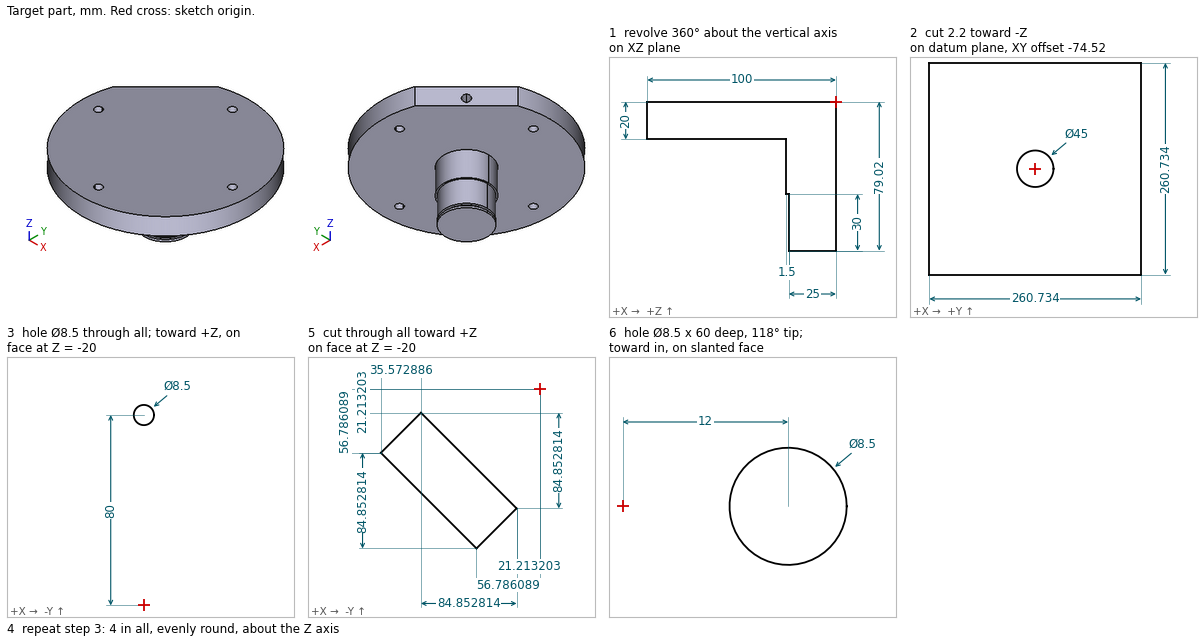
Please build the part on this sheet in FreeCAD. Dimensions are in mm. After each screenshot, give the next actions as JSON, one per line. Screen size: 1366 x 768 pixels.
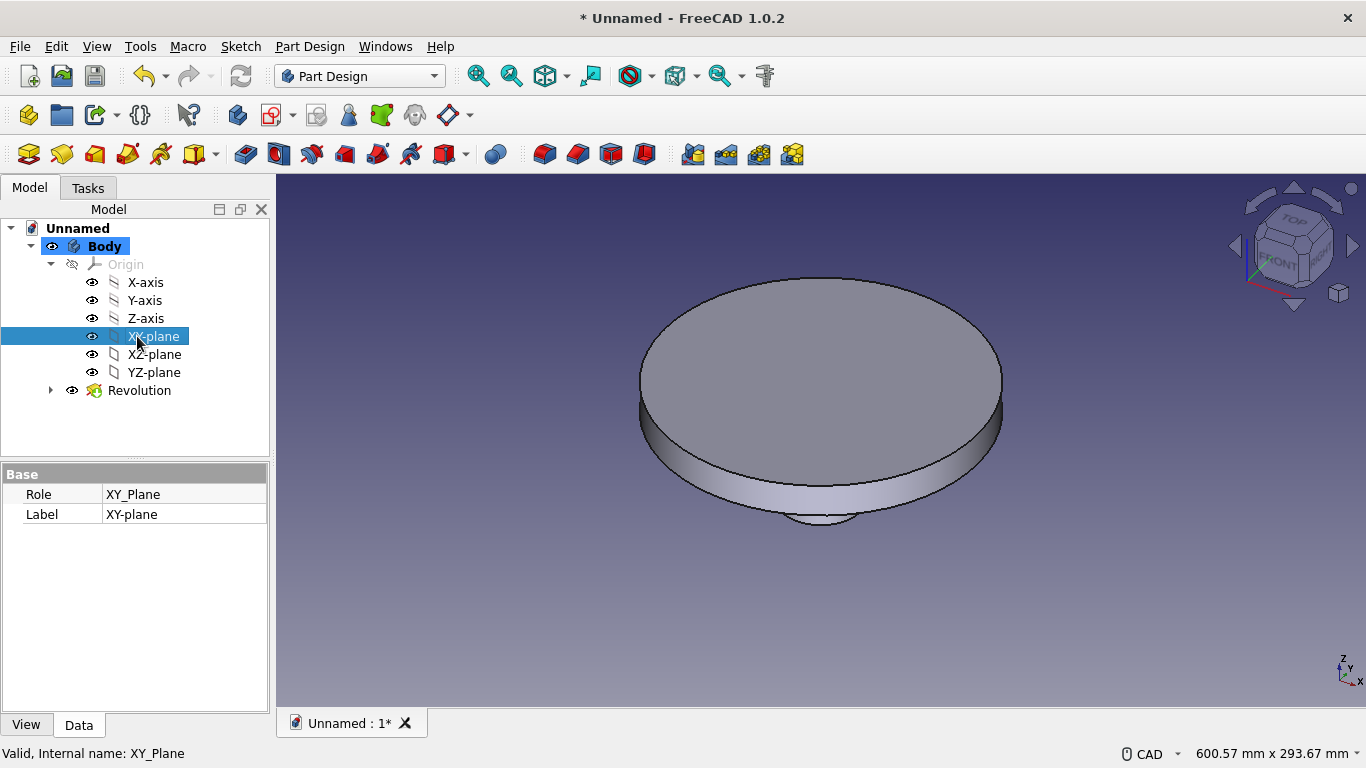
{"action": "left_click", "coordinate": [448, 116]}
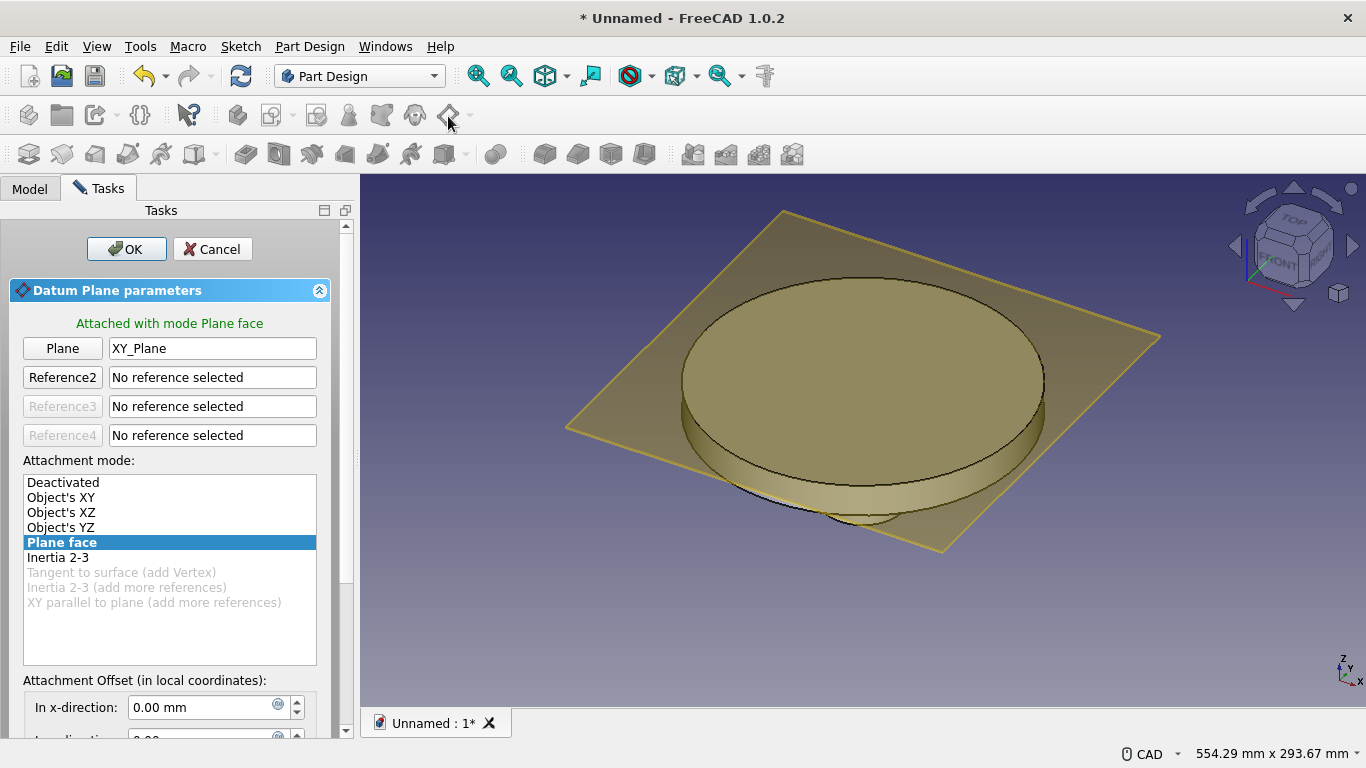
{"action": "scroll", "coordinate": [346, 479], "scroll_direction": "down", "scroll_amount": 2}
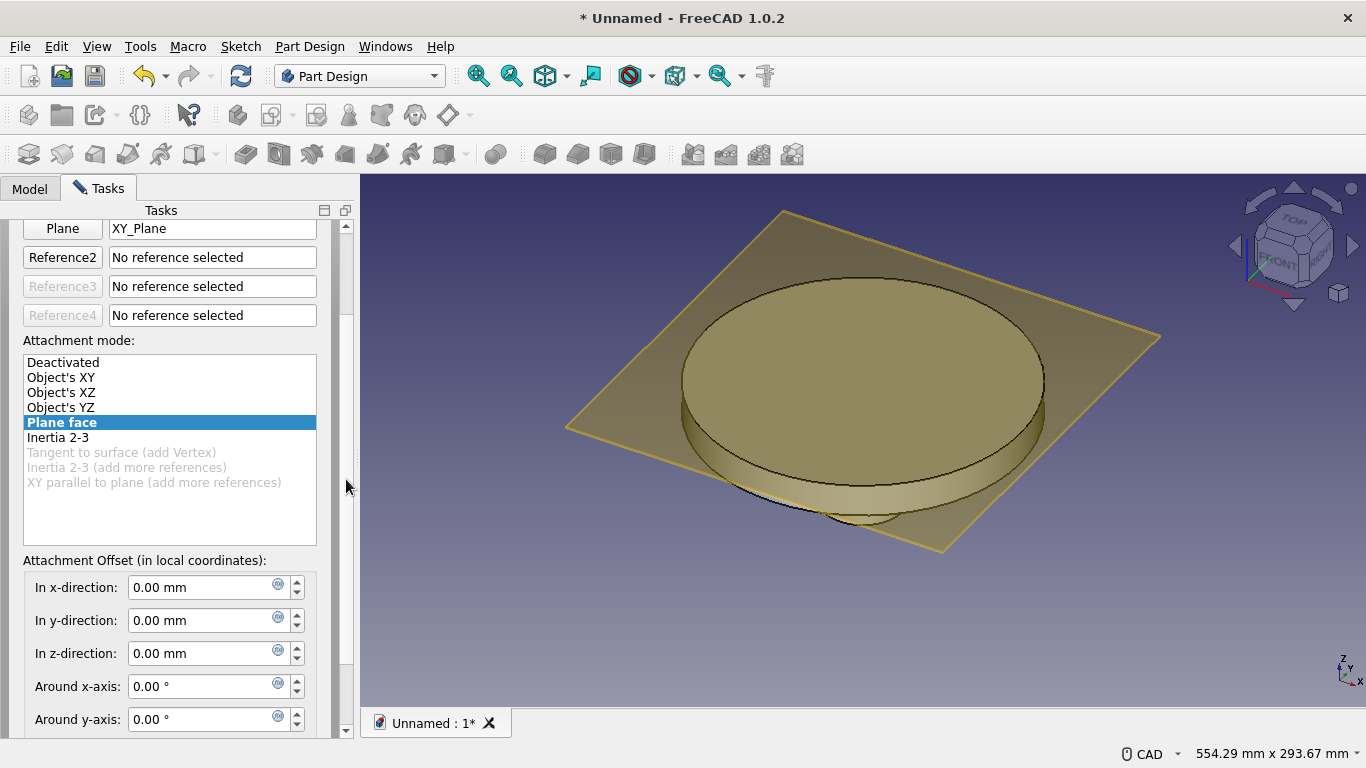
{"action": "triple_click", "coordinate": [210, 654]}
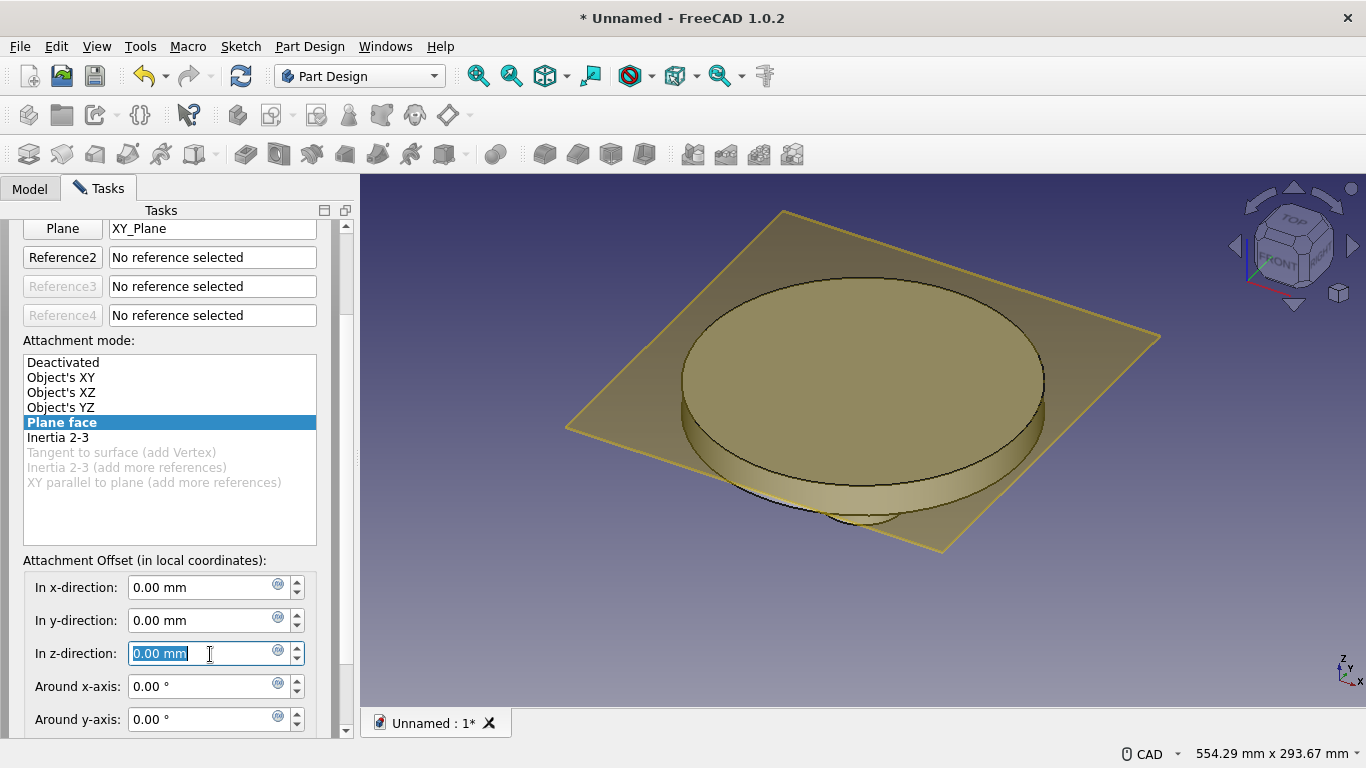
{"action": "type", "text": "-74.52"}
{"action": "key", "text": "Tab"}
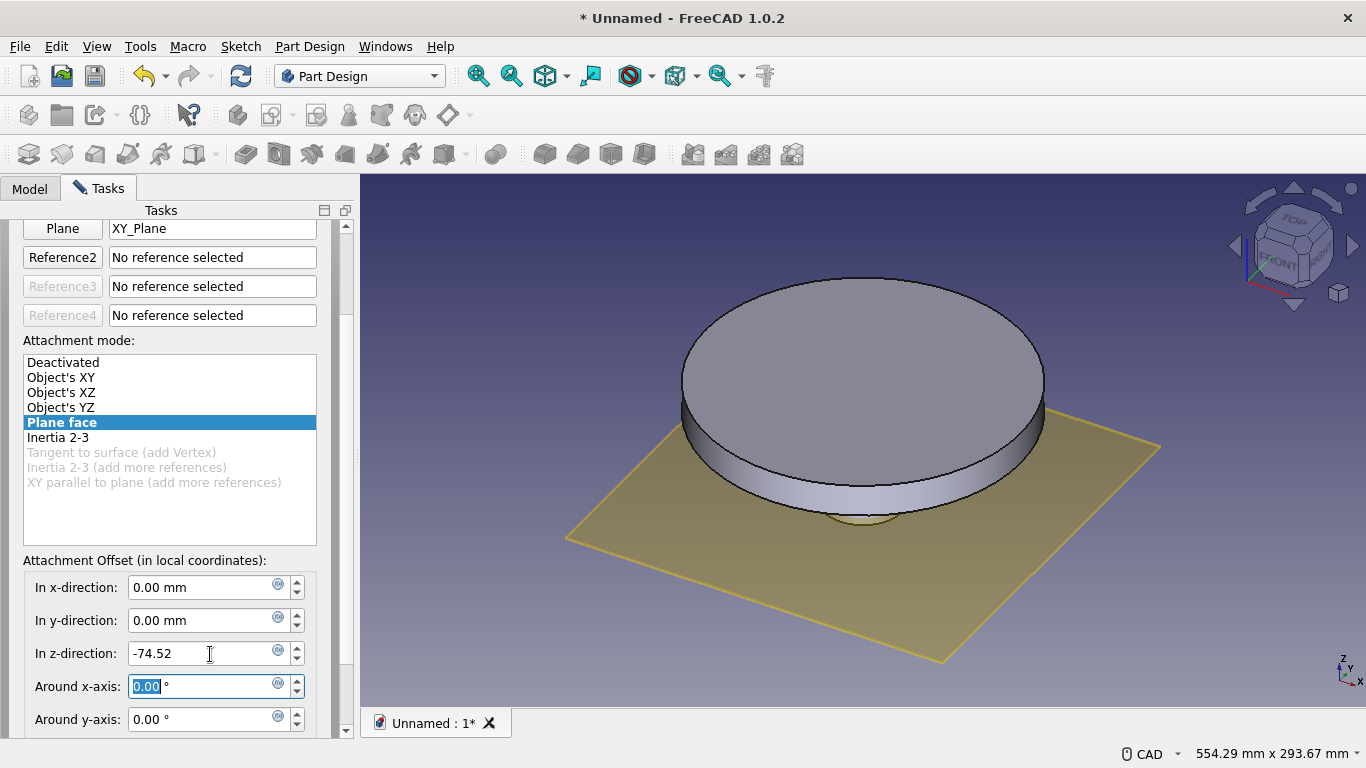
{"action": "scroll", "coordinate": [346, 479], "scroll_direction": "up", "scroll_amount": 3}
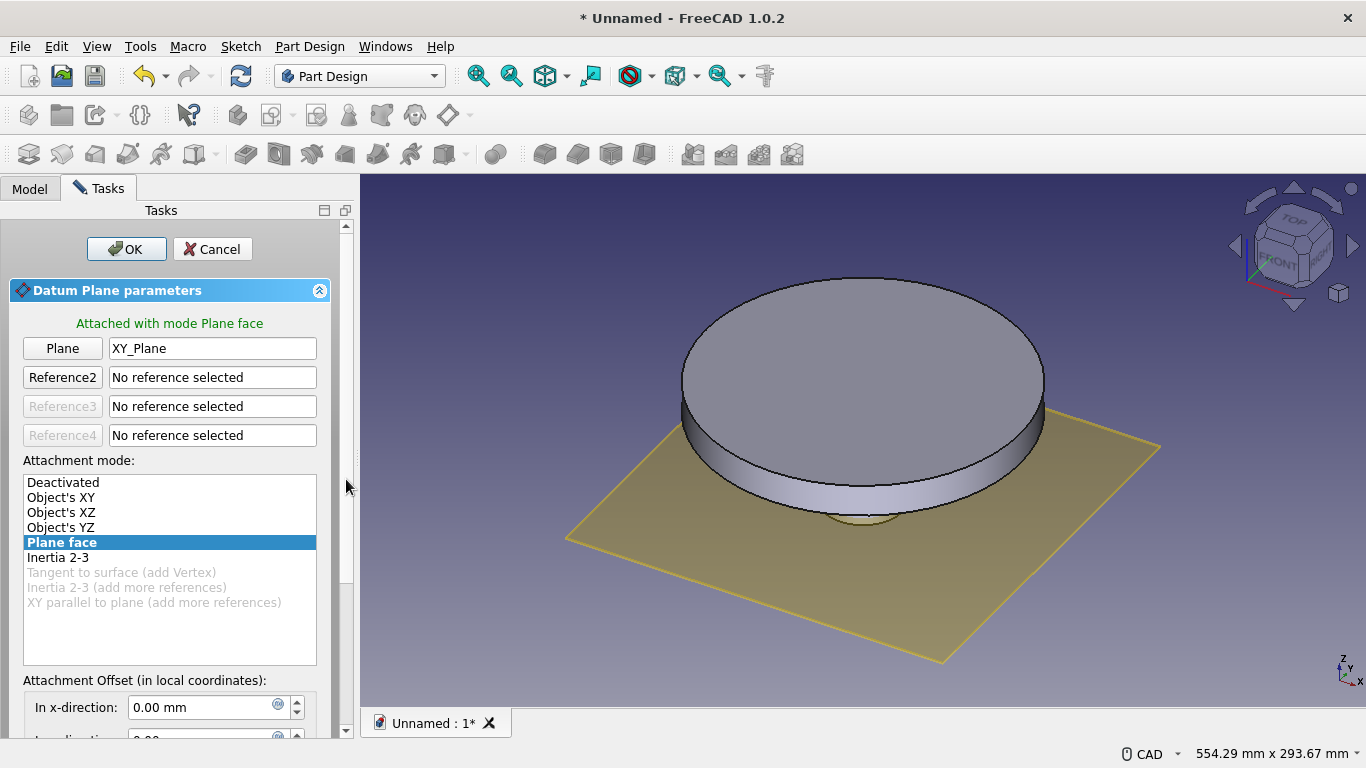
{"action": "left_click", "coordinate": [127, 249]}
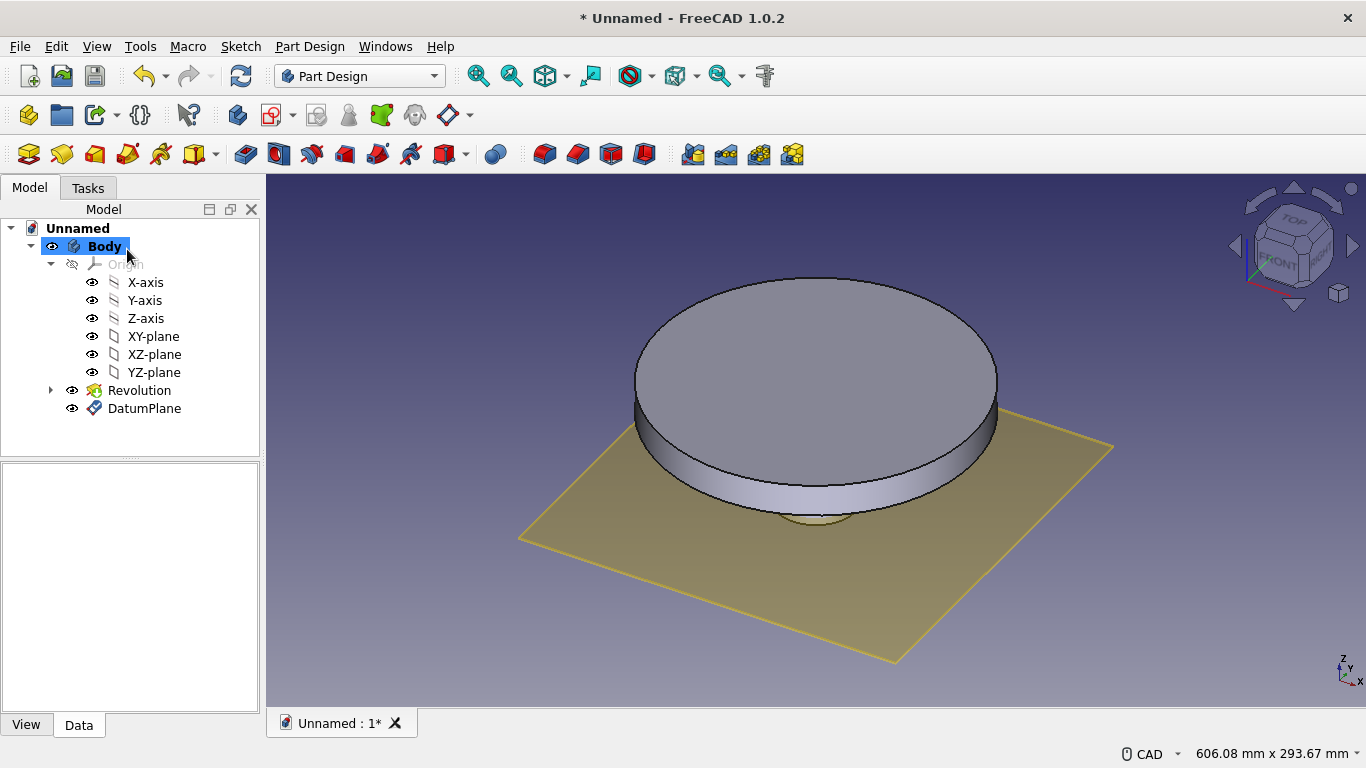
{"action": "left_click", "coordinate": [117, 408]}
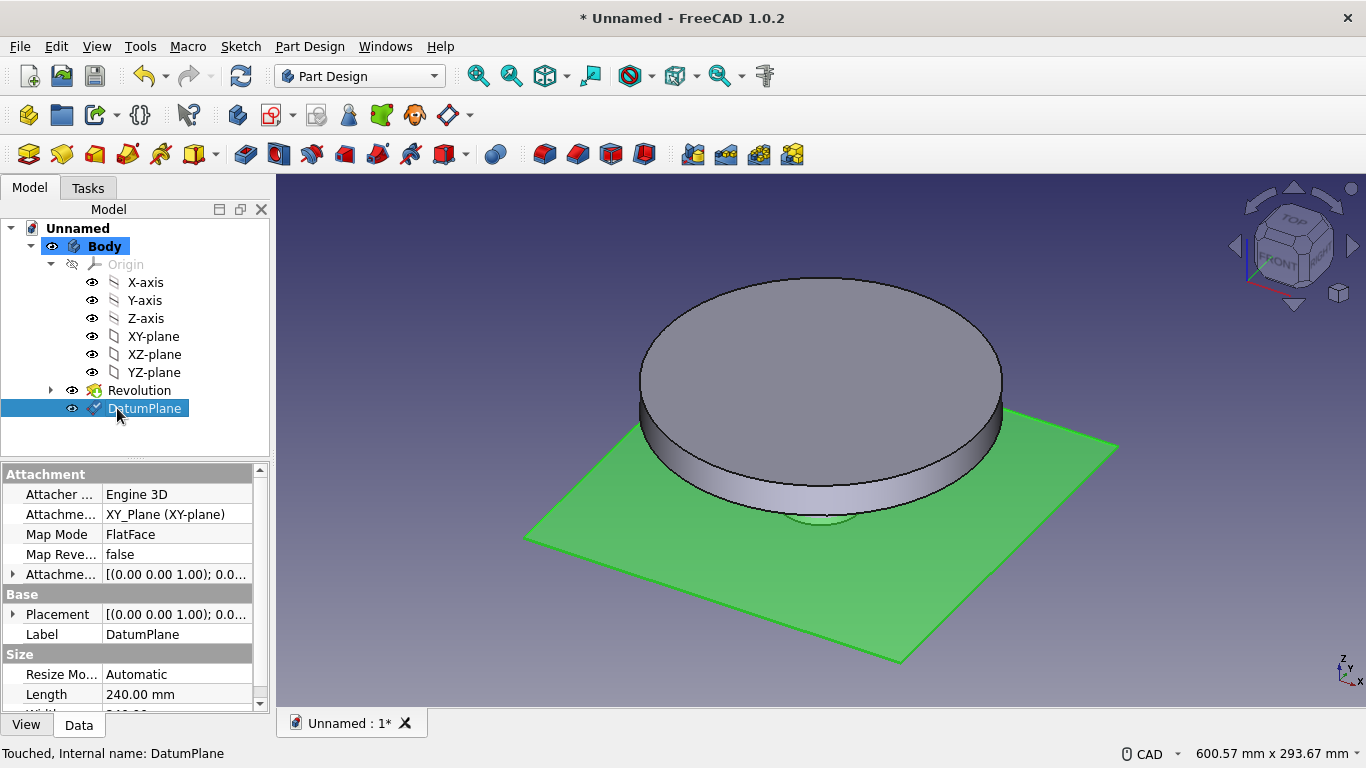
{"action": "left_click", "coordinate": [270, 116]}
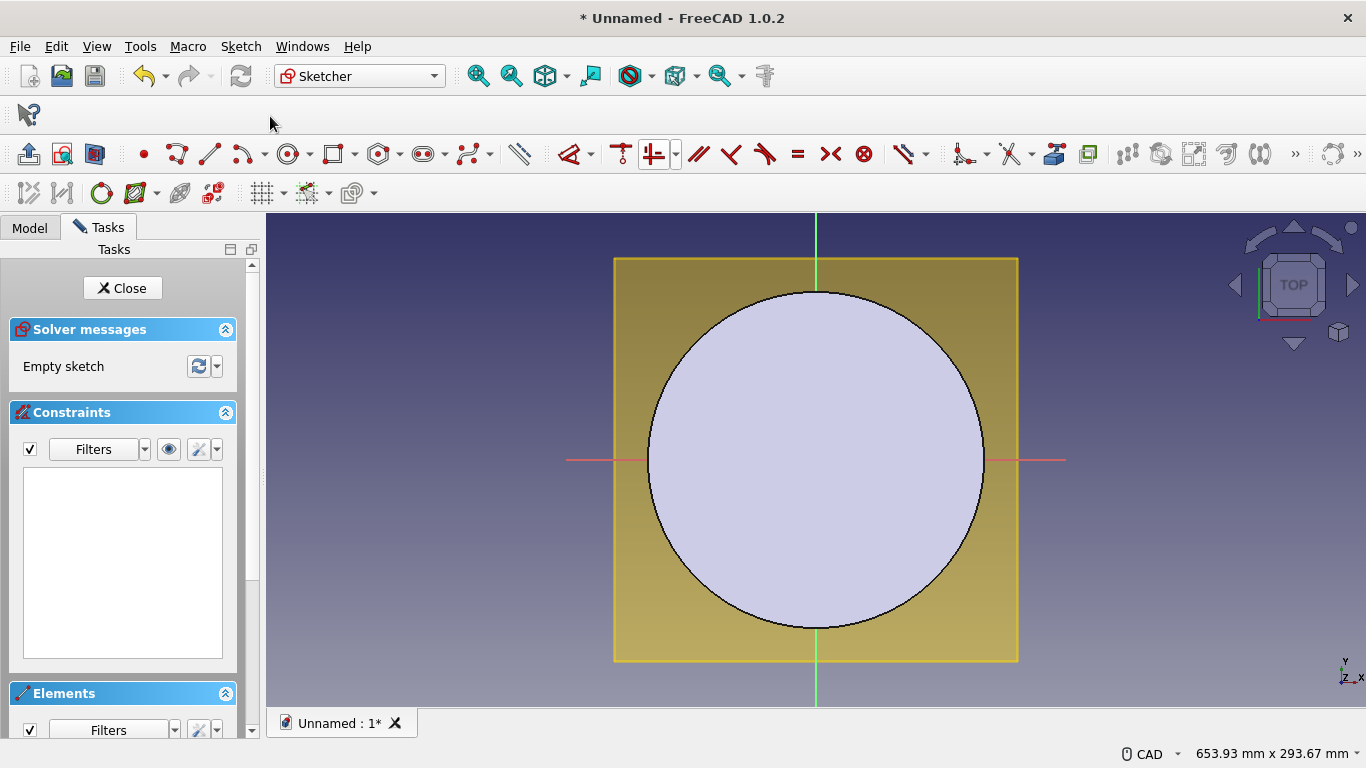
{"action": "left_click", "coordinate": [95, 154]}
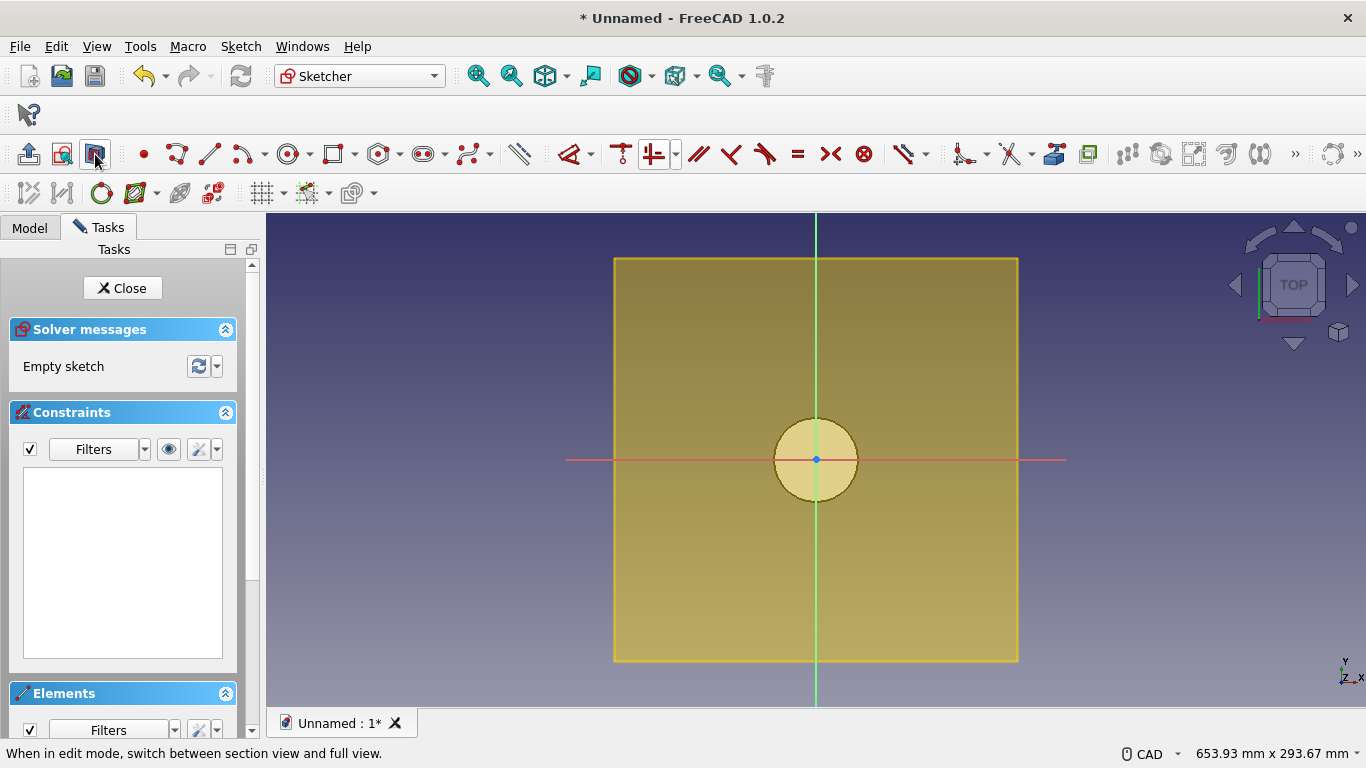
{"action": "scroll", "coordinate": [608, 460], "scroll_direction": "down", "scroll_amount": 2}